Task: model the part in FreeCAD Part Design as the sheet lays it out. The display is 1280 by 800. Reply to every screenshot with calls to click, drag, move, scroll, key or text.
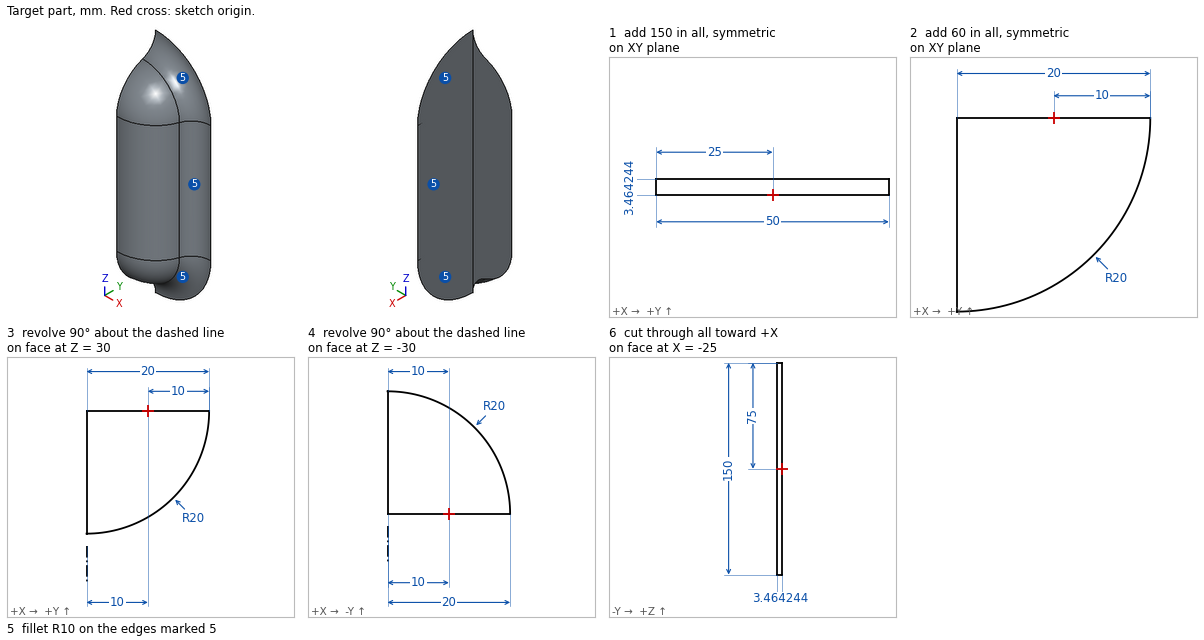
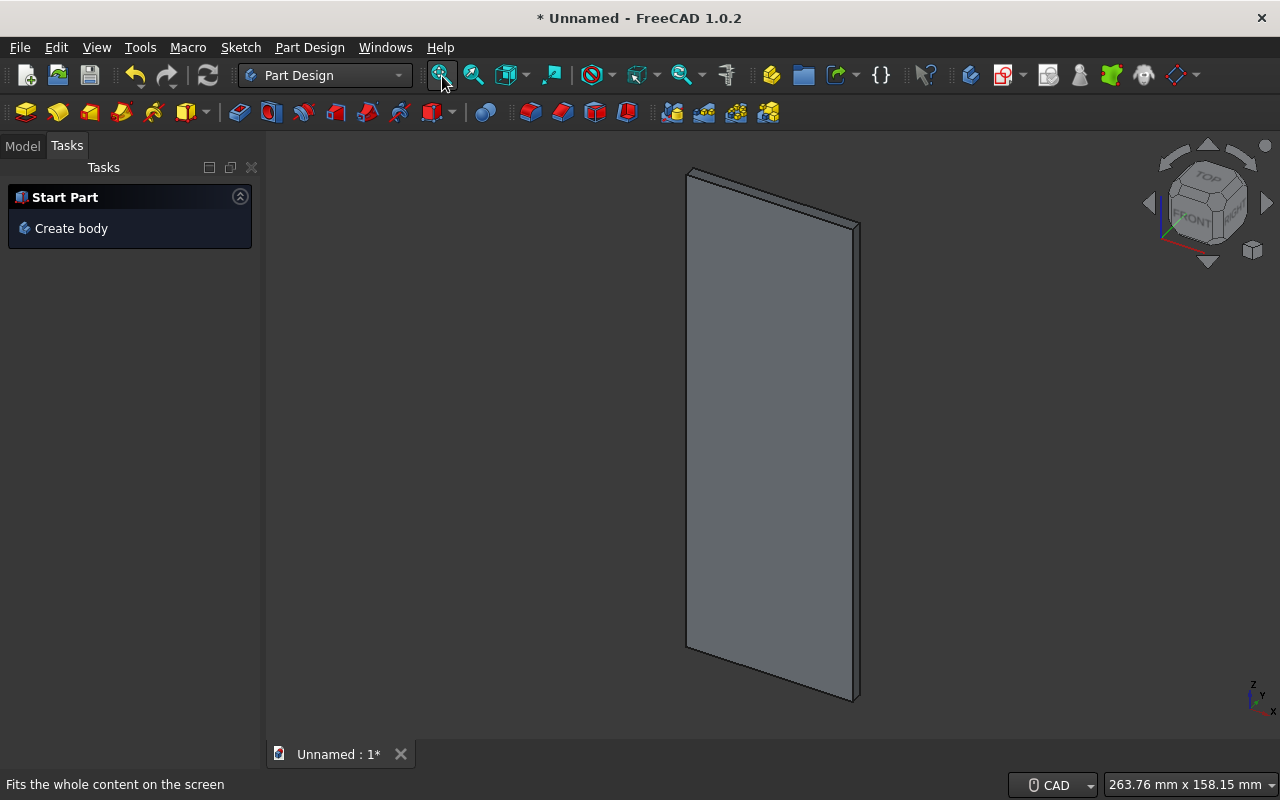
click(1004, 76)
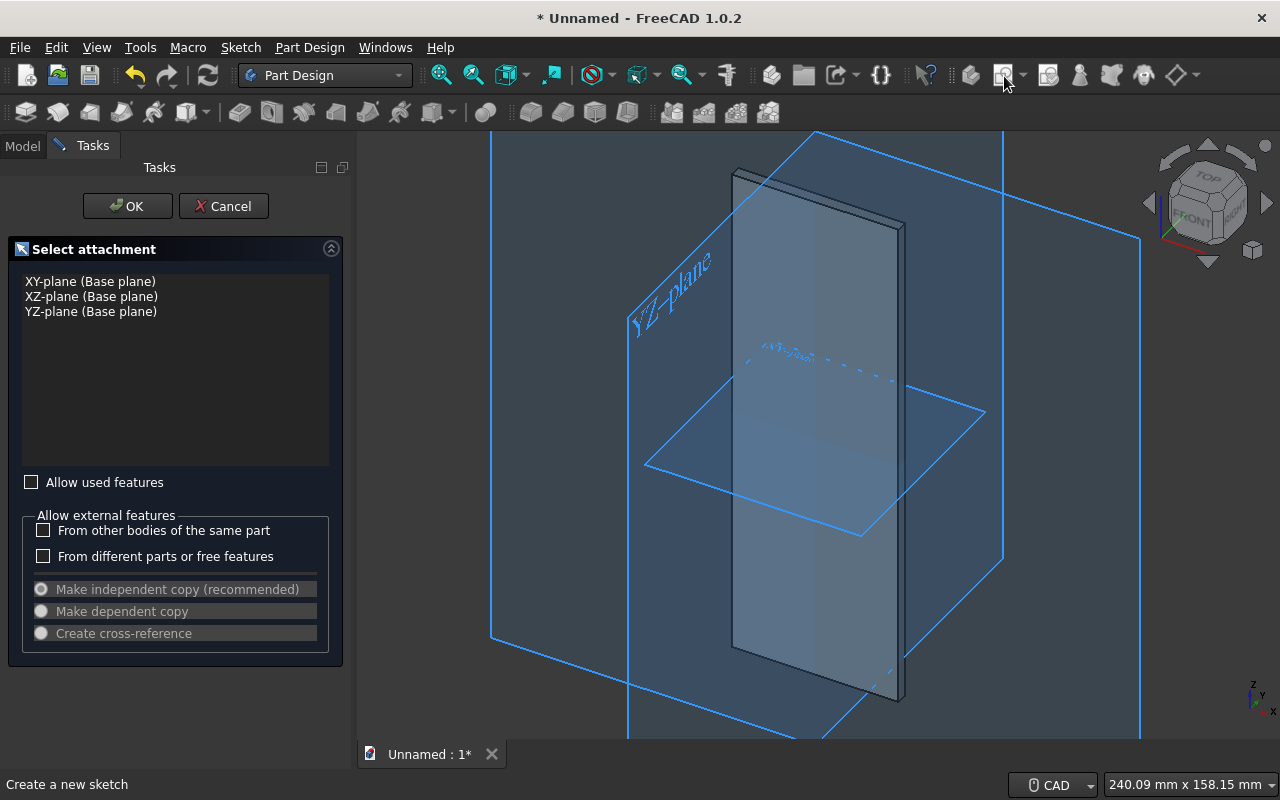
click(82, 282)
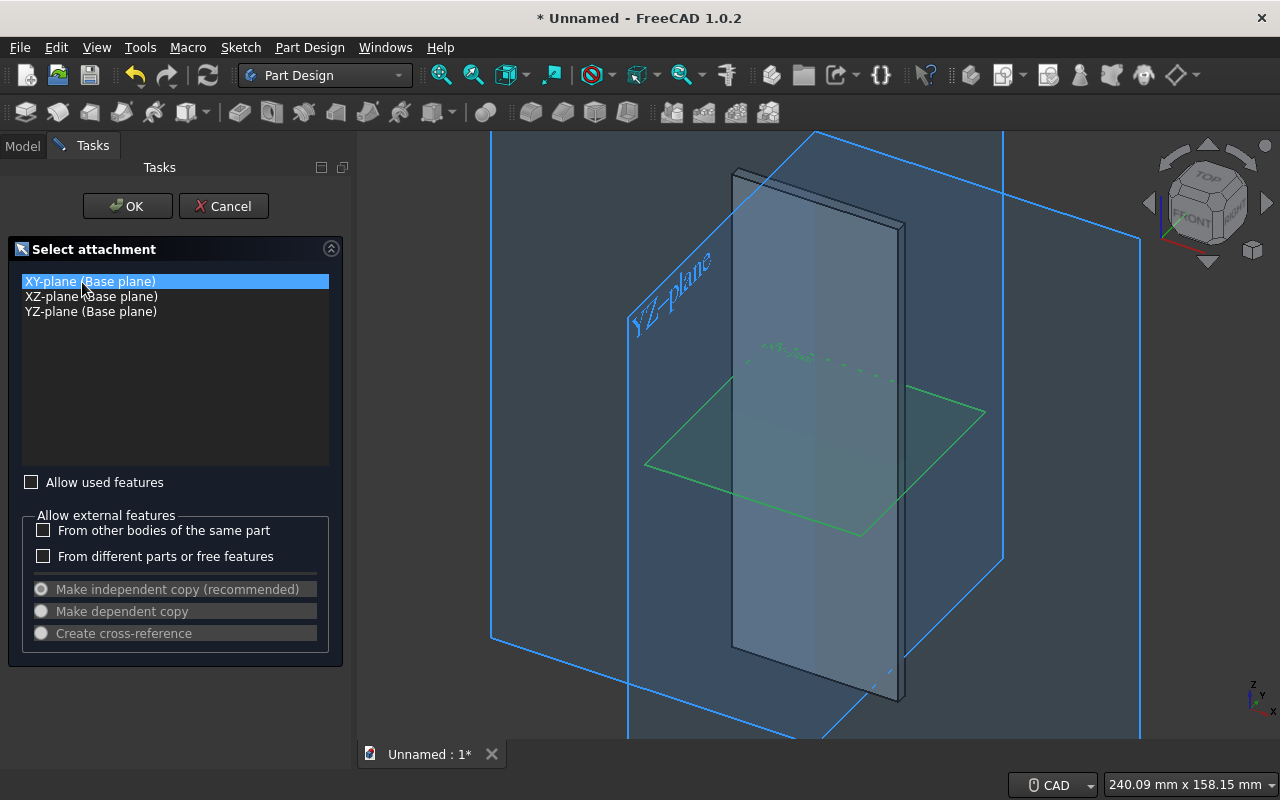
click(128, 206)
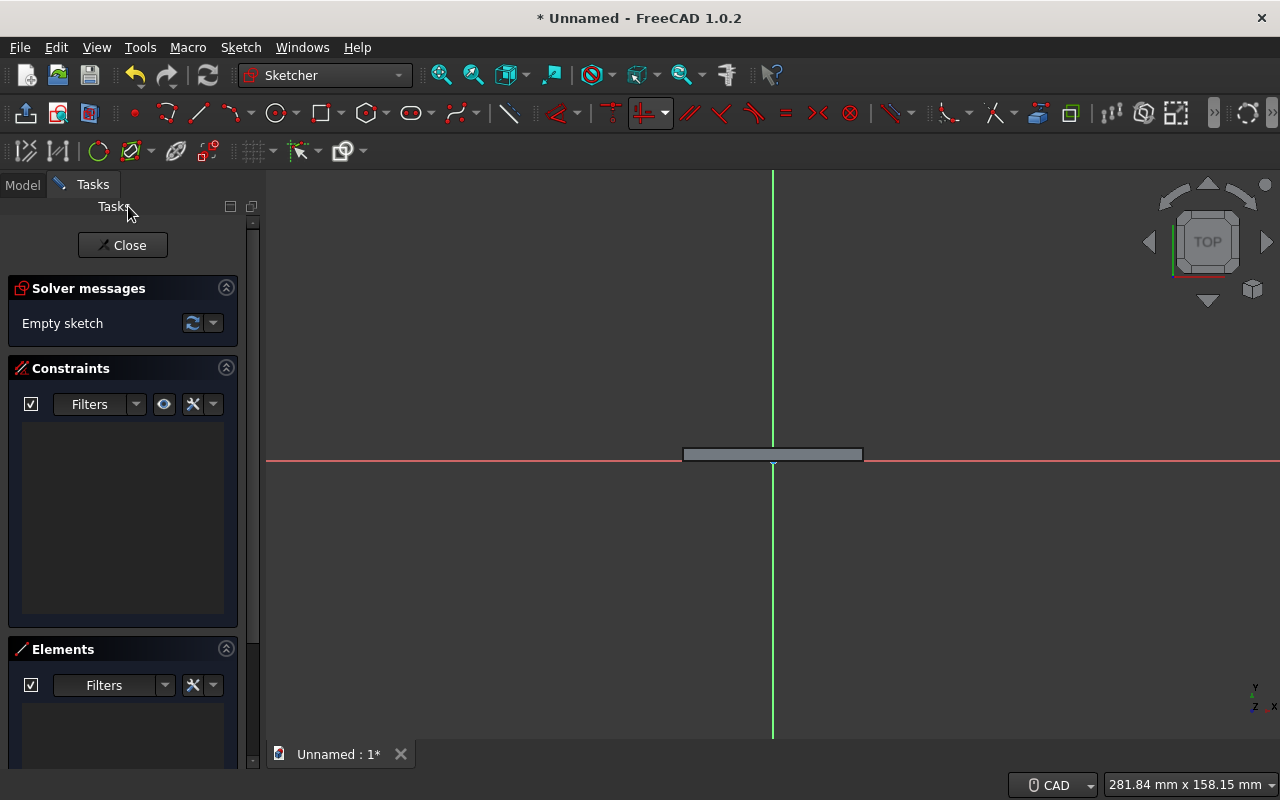
click(90, 114)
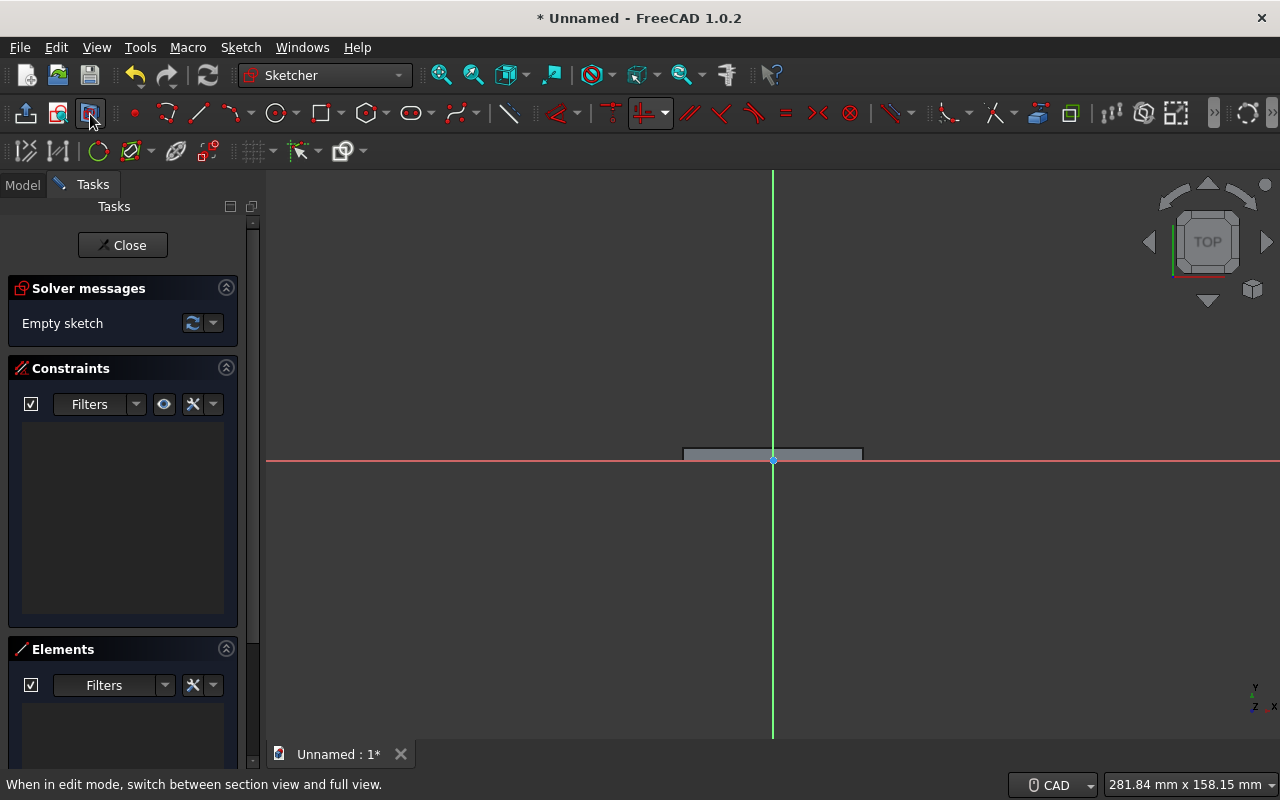
scroll(790, 507, up, 8)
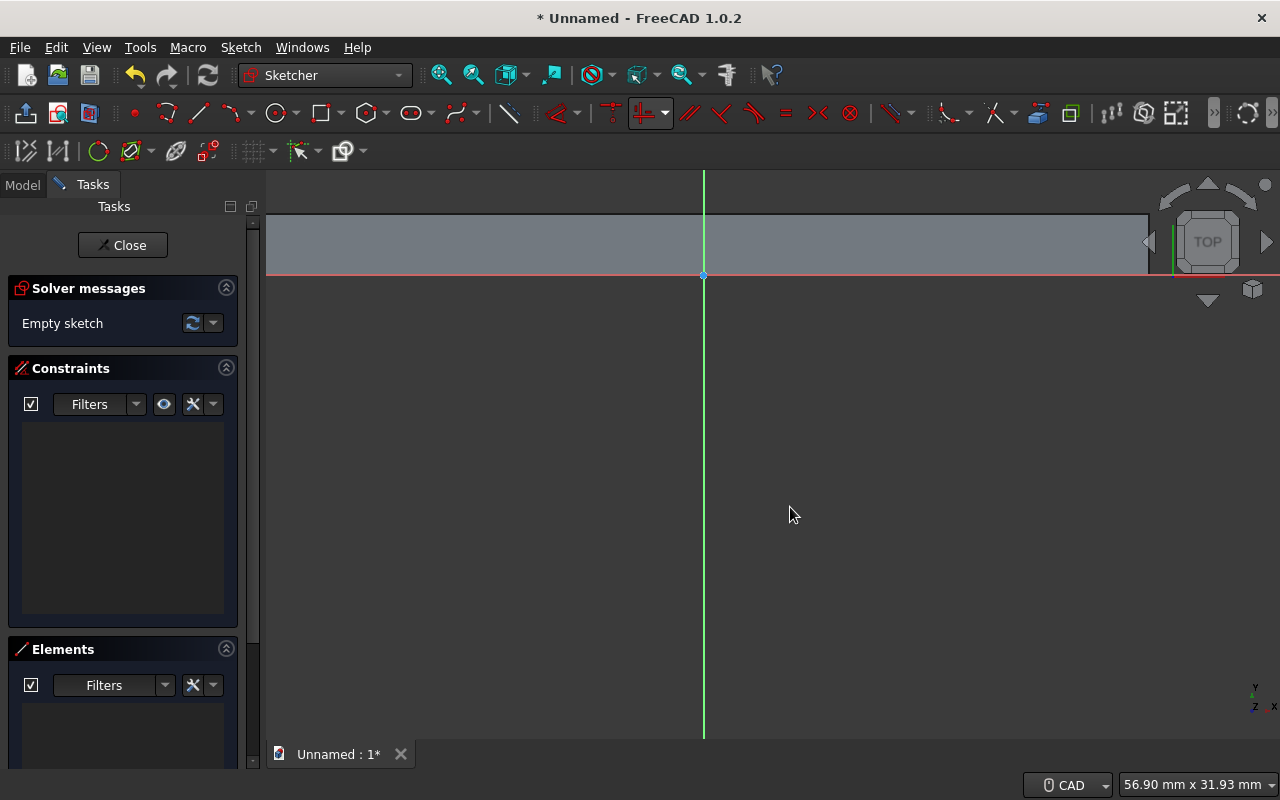
click(168, 114)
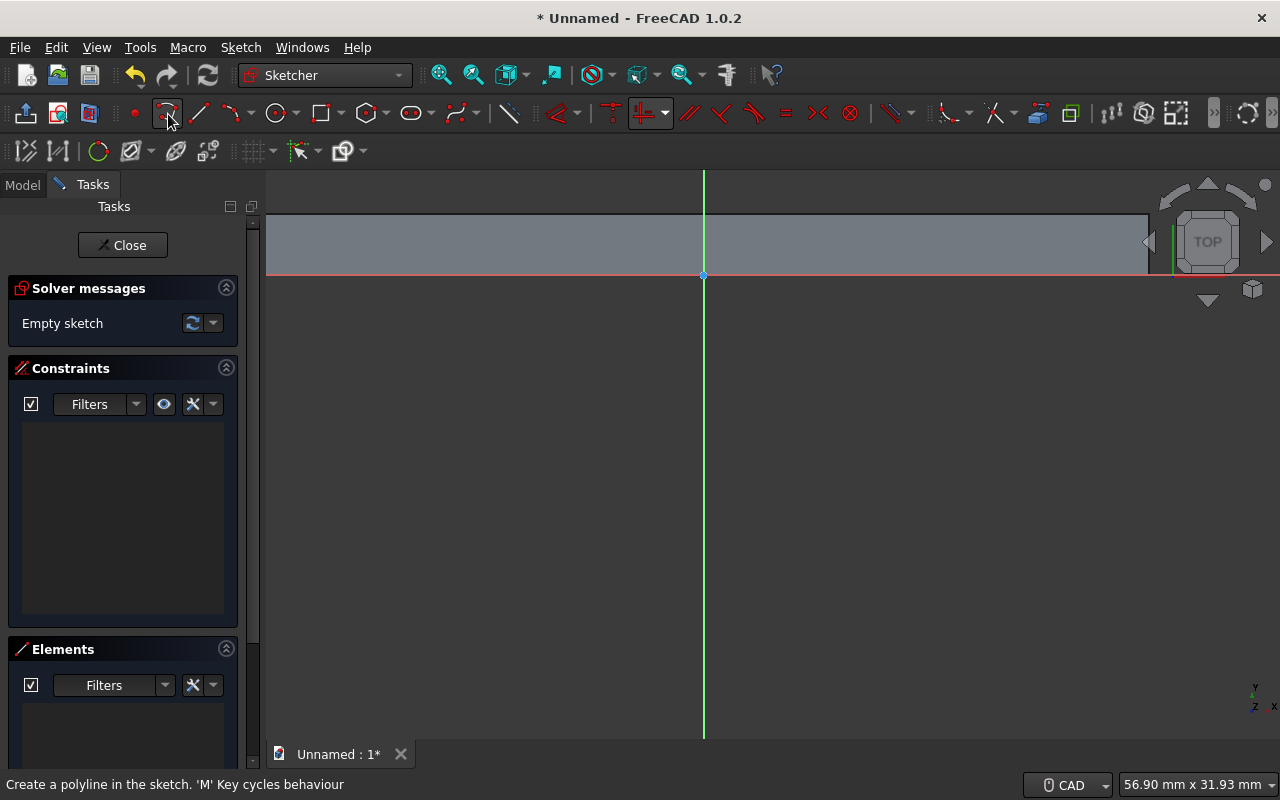
click(882, 275)
click(526, 284)
click(526, 632)
right_click(526, 632)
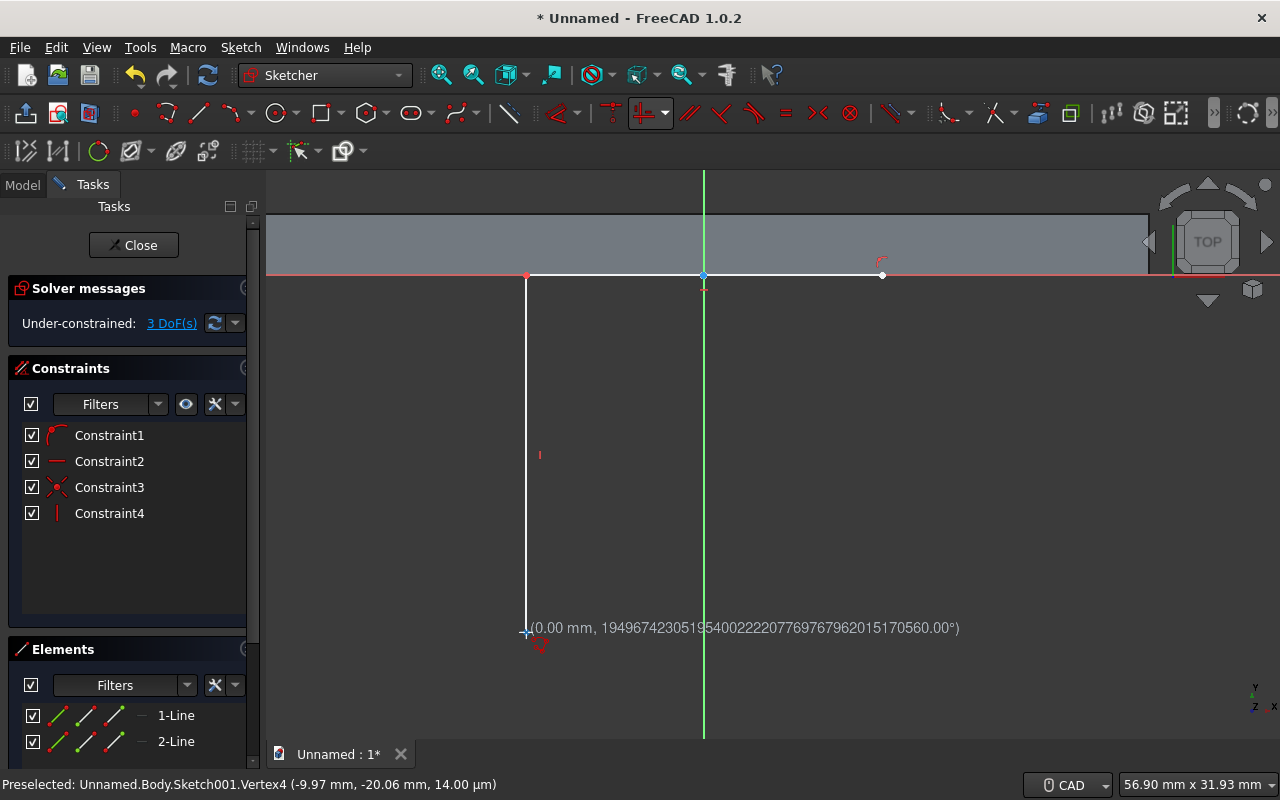
click(232, 114)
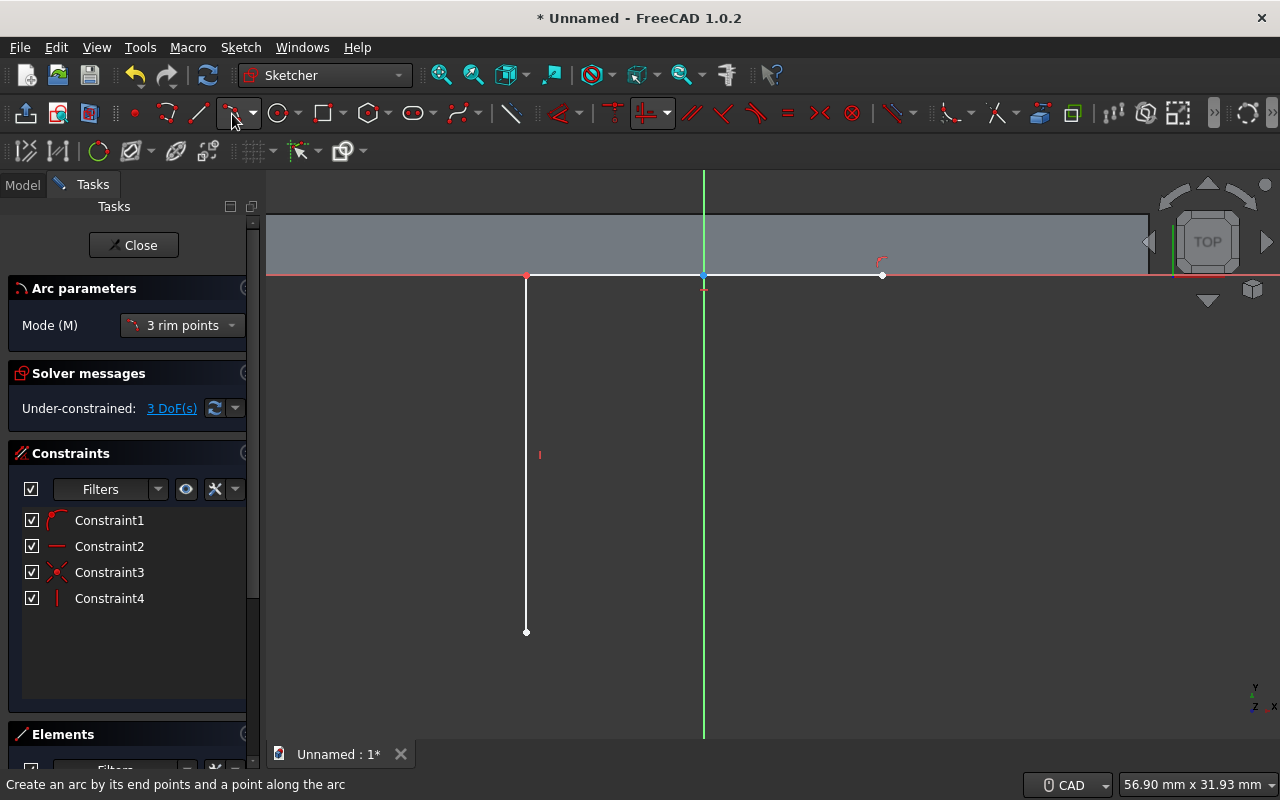
click(526, 633)
click(882, 275)
click(778, 528)
key(Escape)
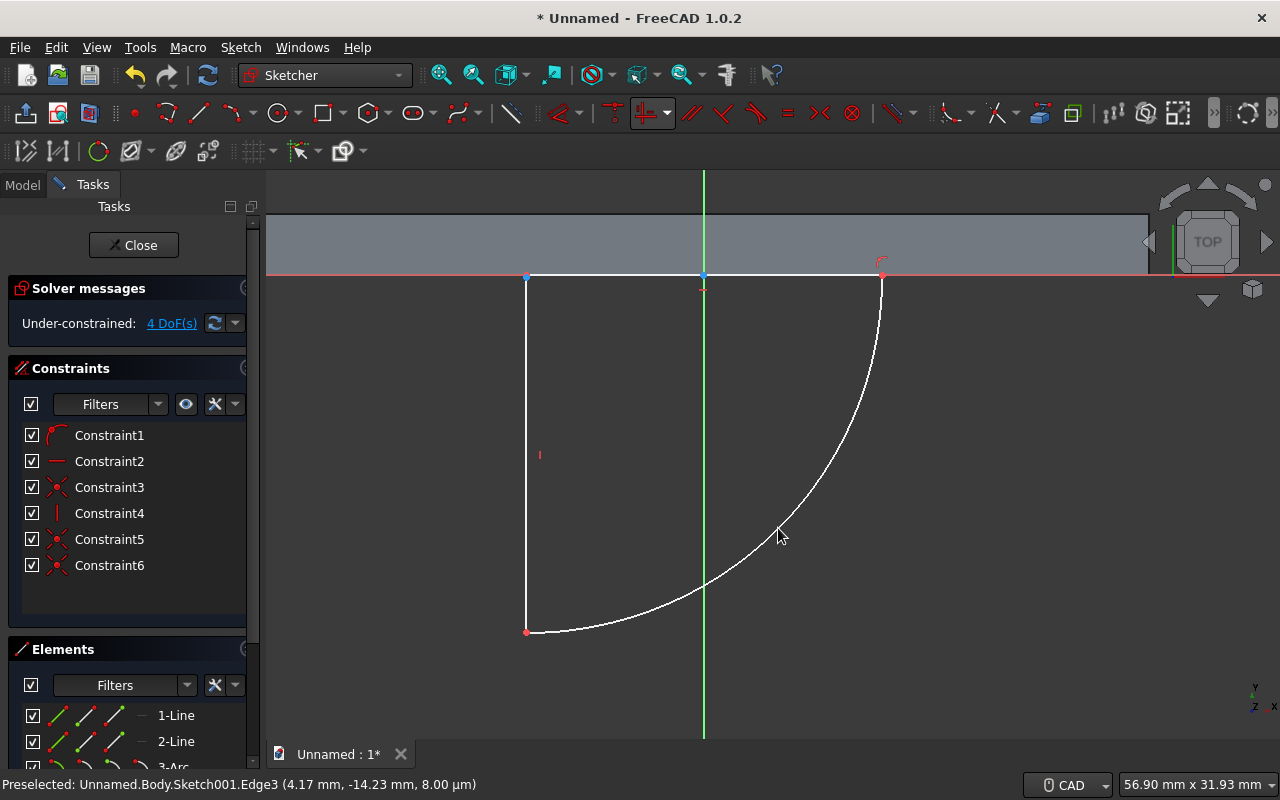
click(527, 278)